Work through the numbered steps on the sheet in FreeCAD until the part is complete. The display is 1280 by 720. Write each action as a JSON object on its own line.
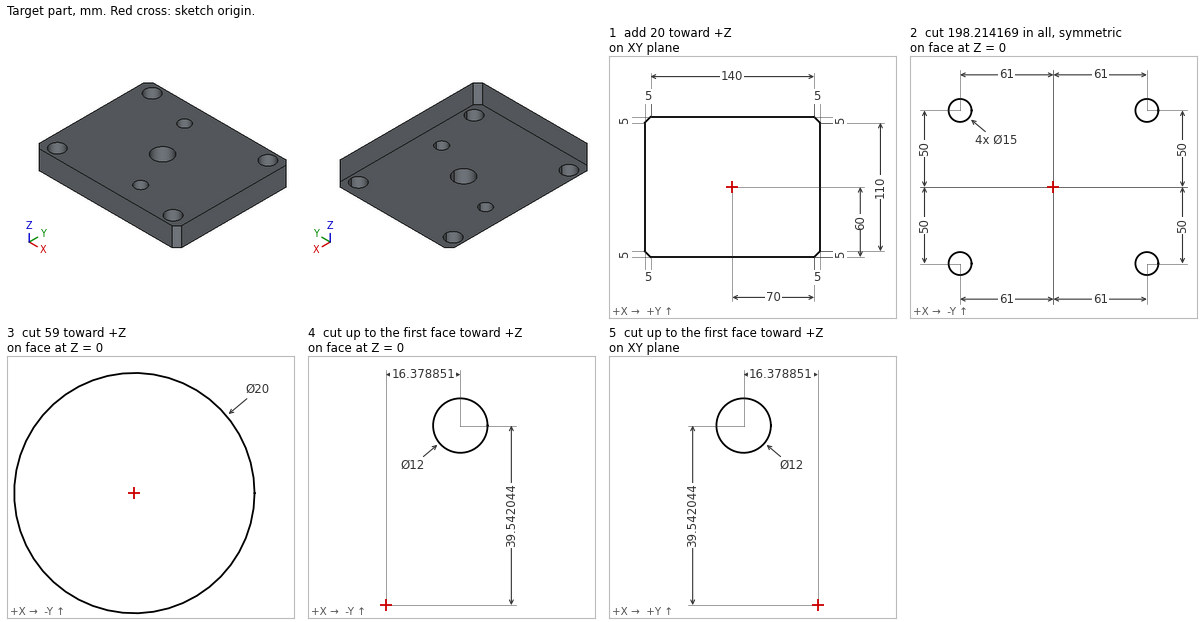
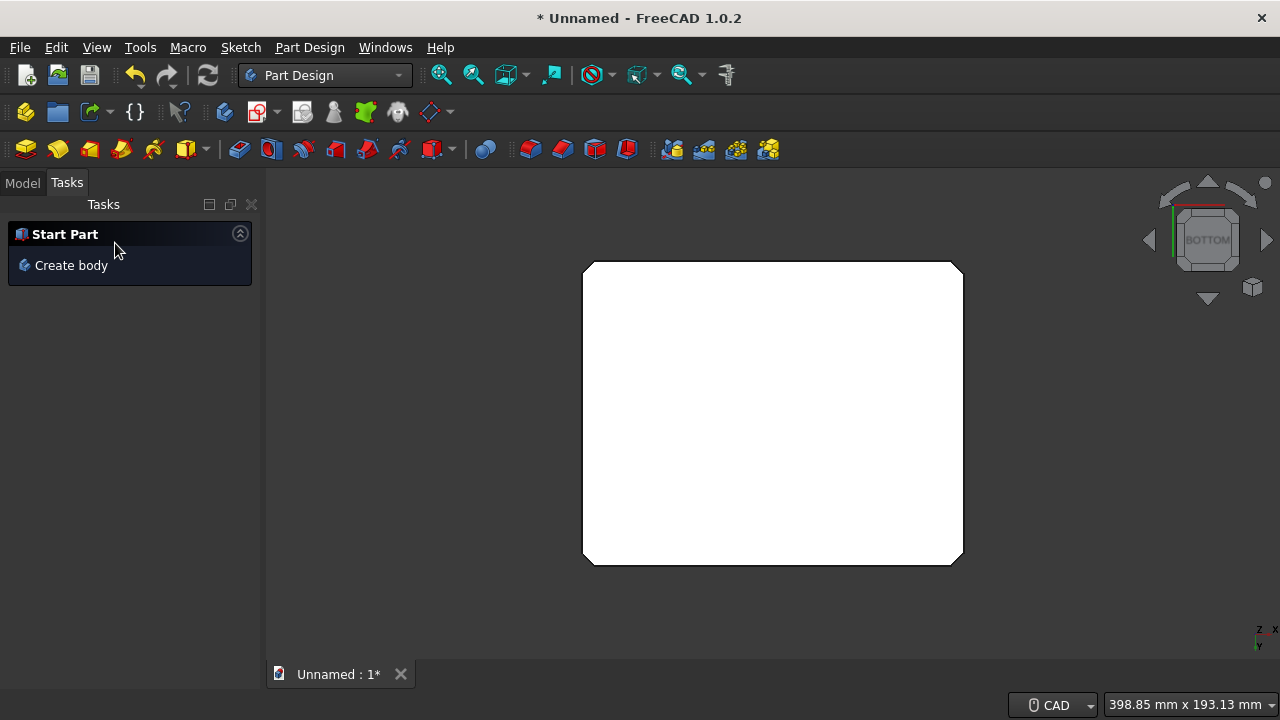
{"action": "left_click", "coordinate": [773, 412]}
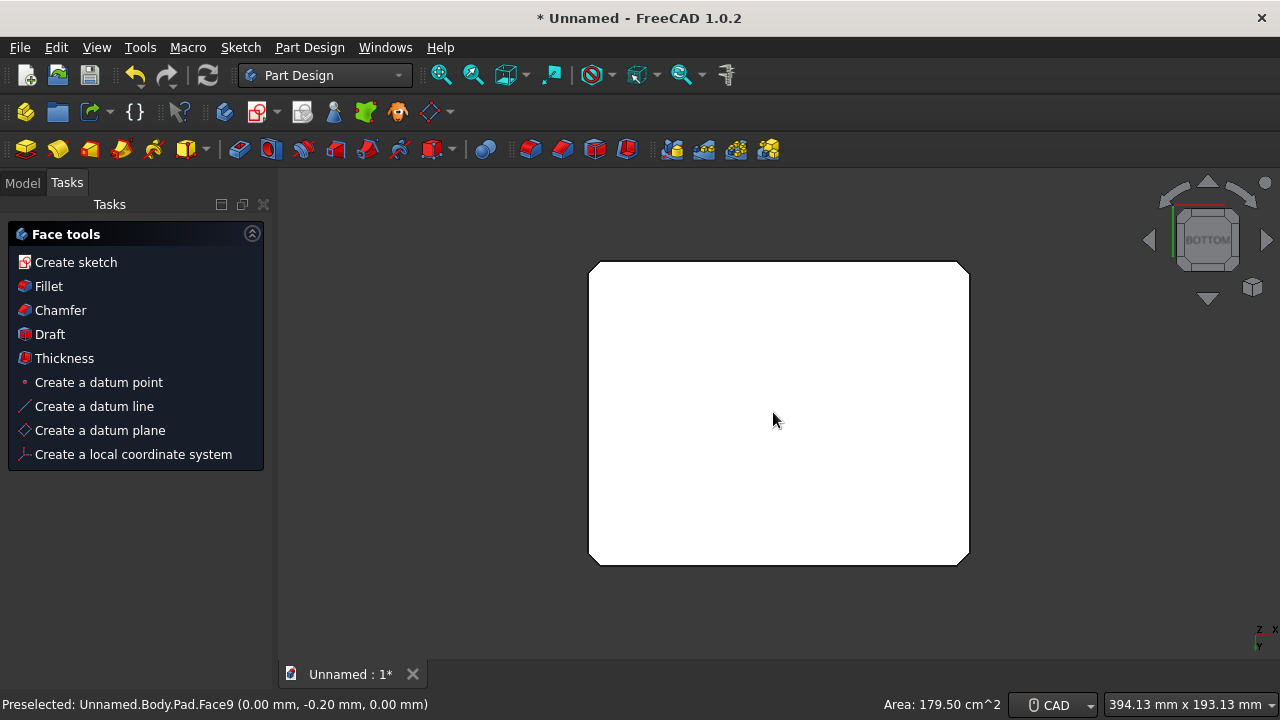
{"action": "left_click", "coordinate": [258, 112]}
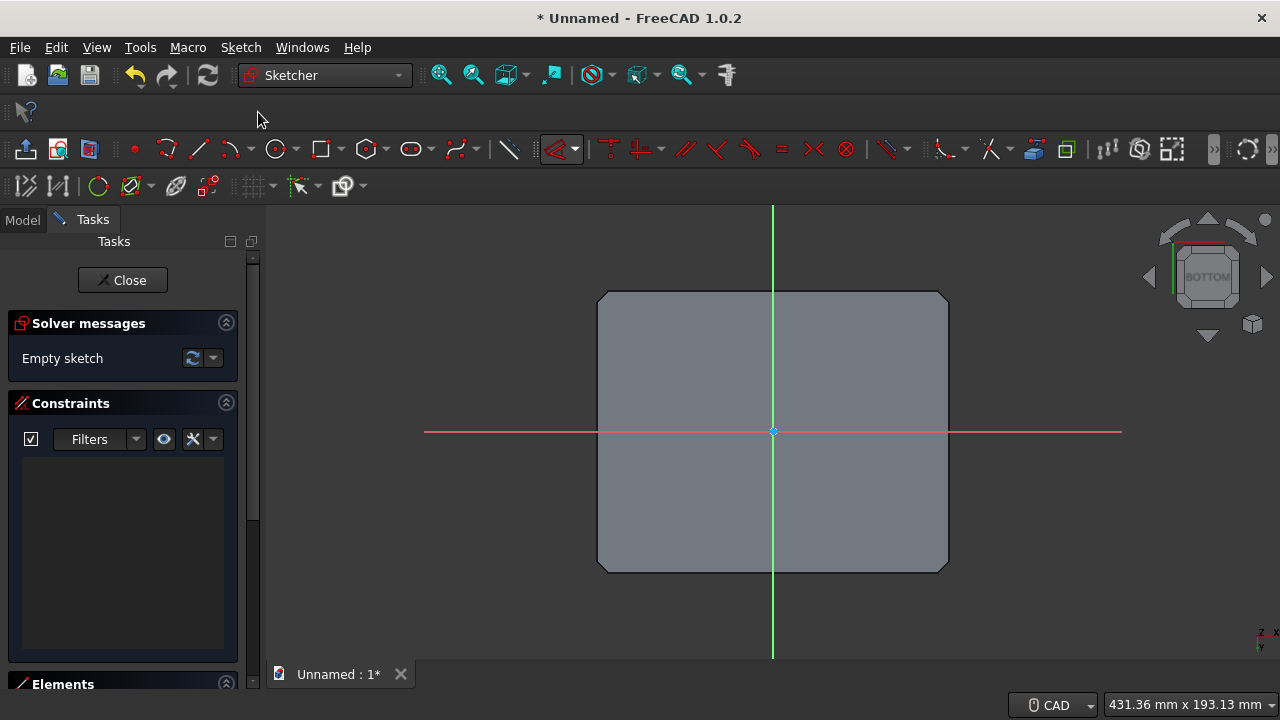
{"action": "key", "text": "g c"}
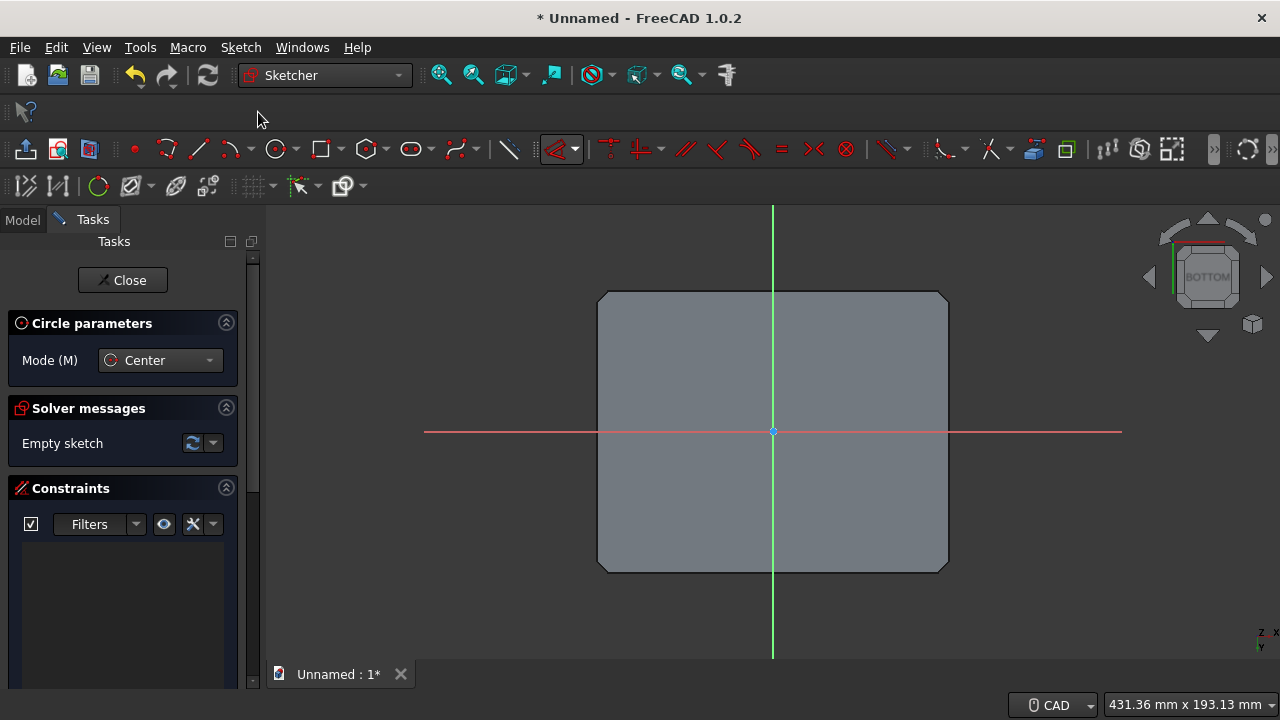
{"action": "scroll", "coordinate": [630, 314], "scroll_direction": "up", "scroll_amount": 2}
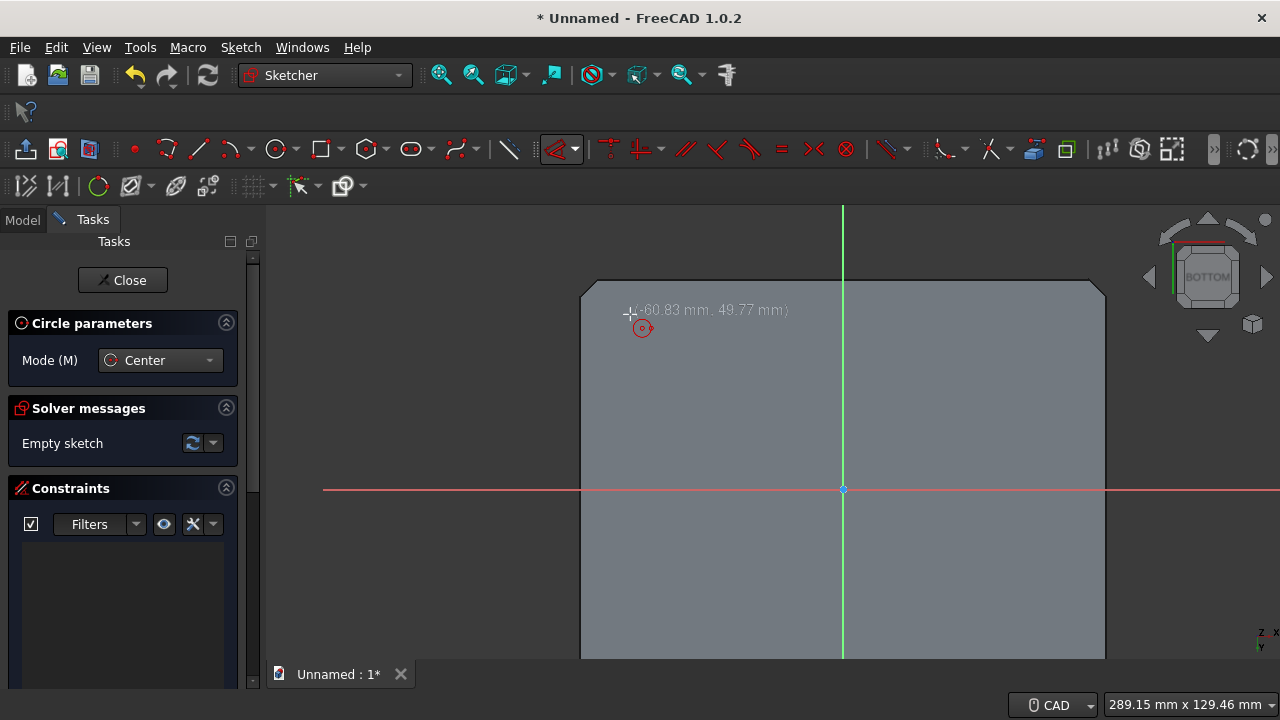
{"action": "left_click", "coordinate": [629, 315]}
{"action": "mouse_move", "coordinate": [648, 296]}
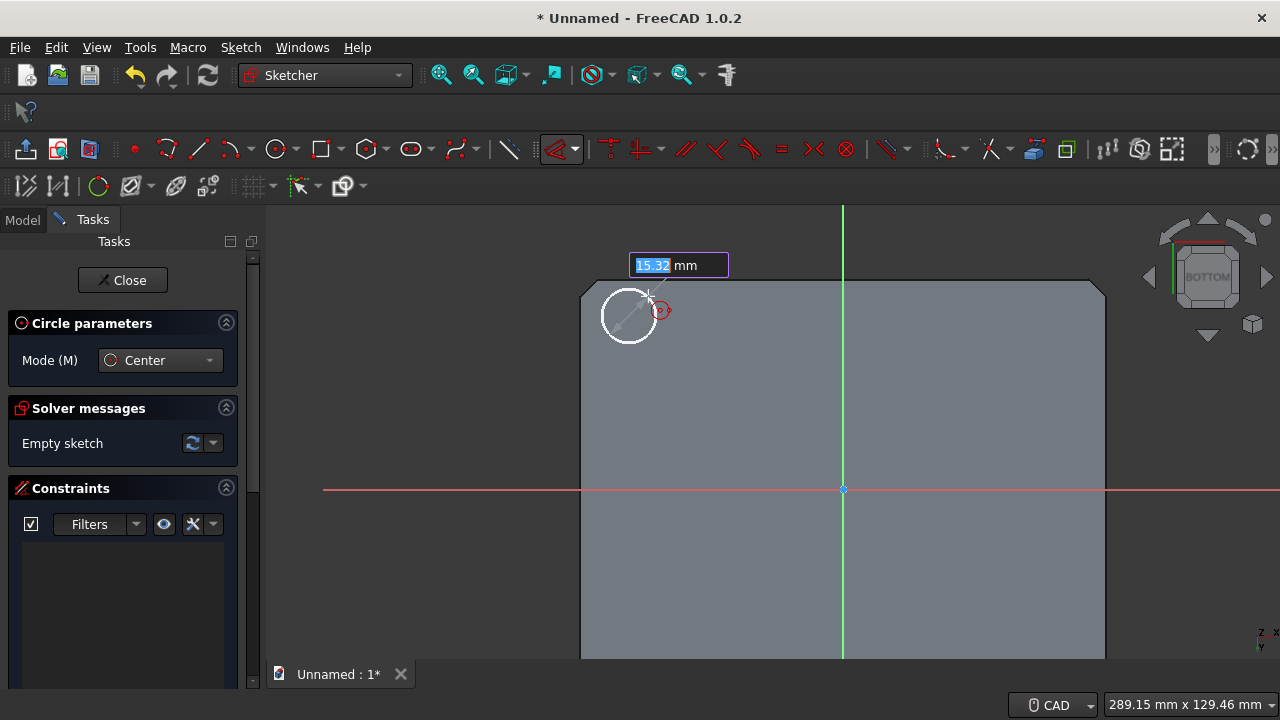
{"action": "type", "text": "15"}
{"action": "key", "text": "Return"}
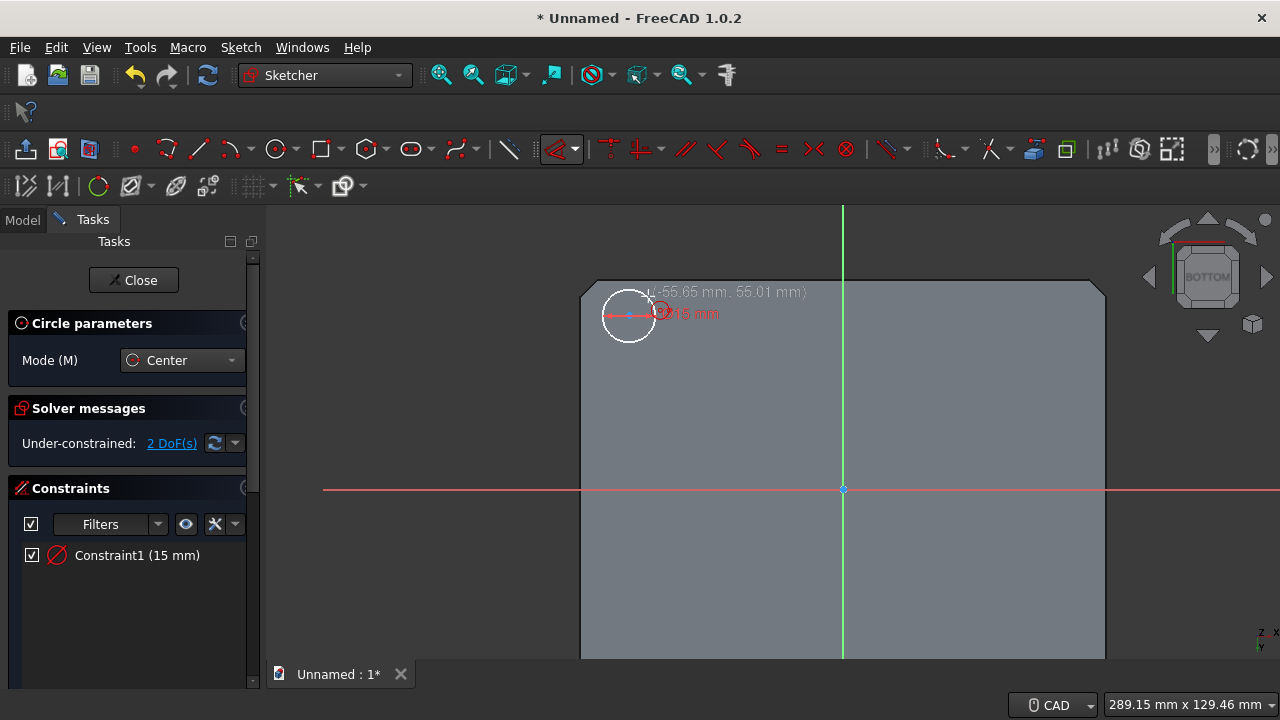
{"action": "scroll", "coordinate": [423, 314], "scroll_direction": "down", "scroll_amount": 2}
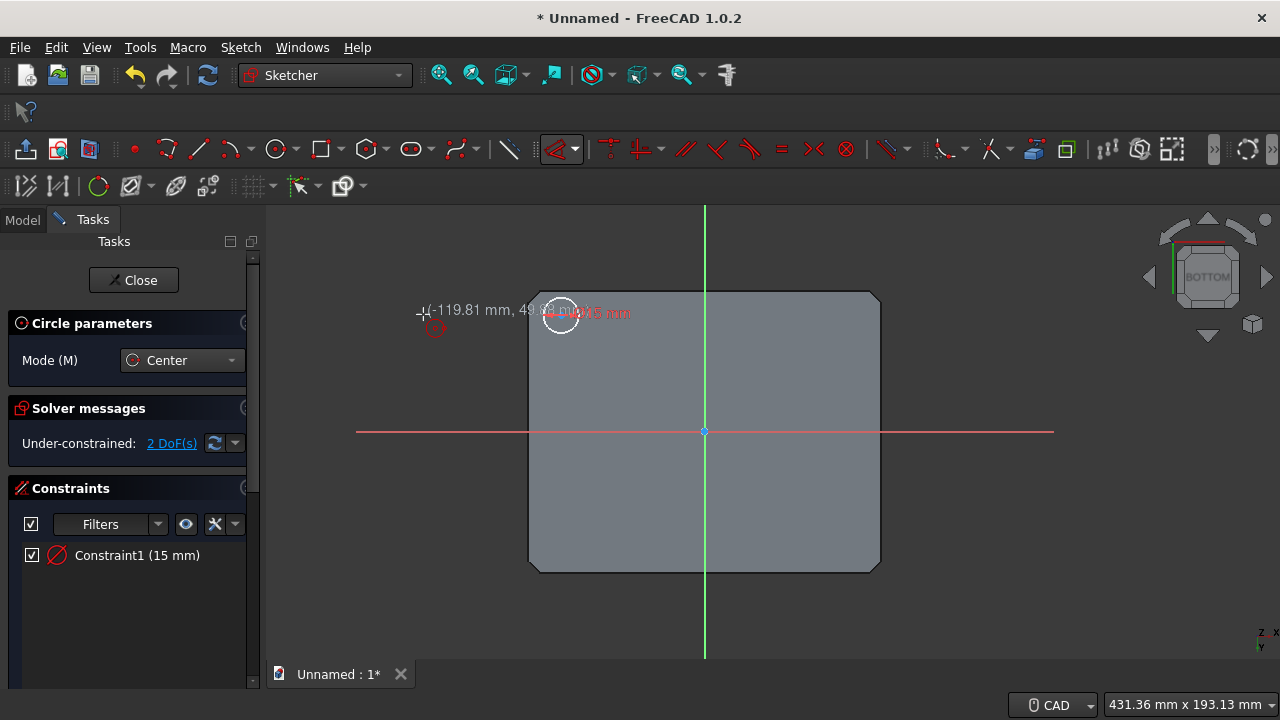
{"action": "scroll", "coordinate": [561, 550], "scroll_direction": "up", "scroll_amount": 2}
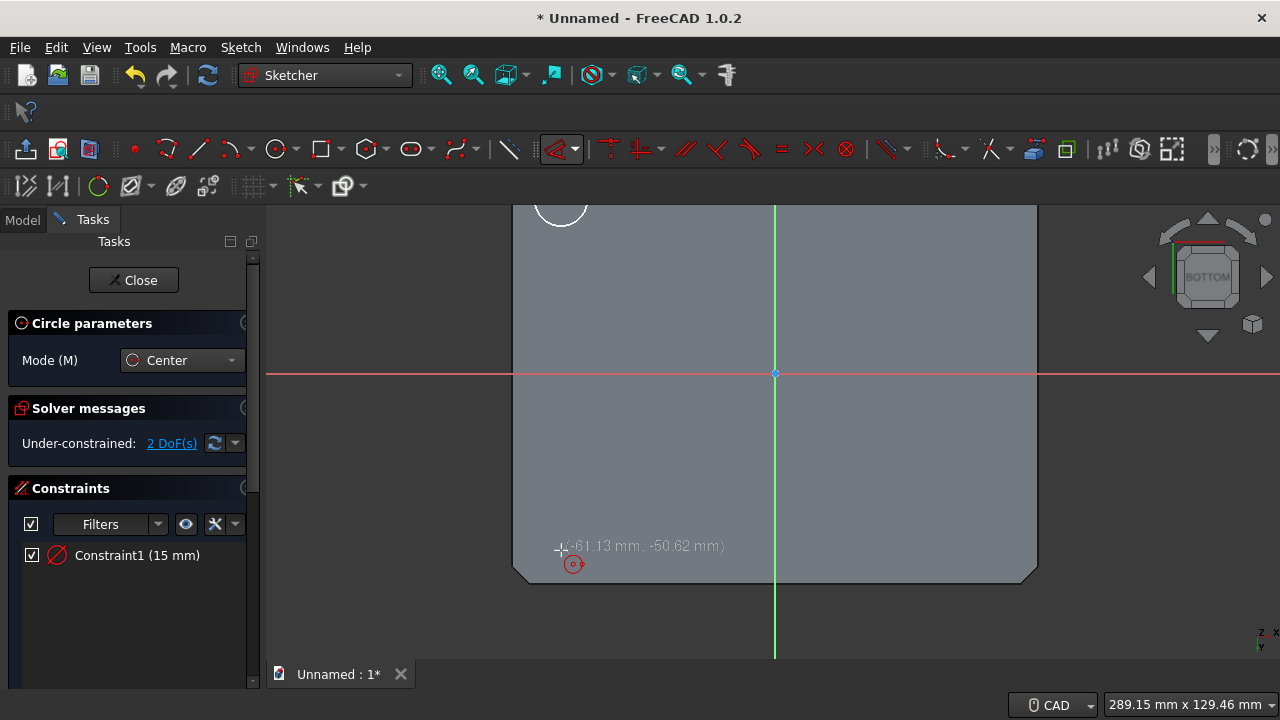
{"action": "left_click", "coordinate": [561, 549]}
{"action": "mouse_move", "coordinate": [580, 530]}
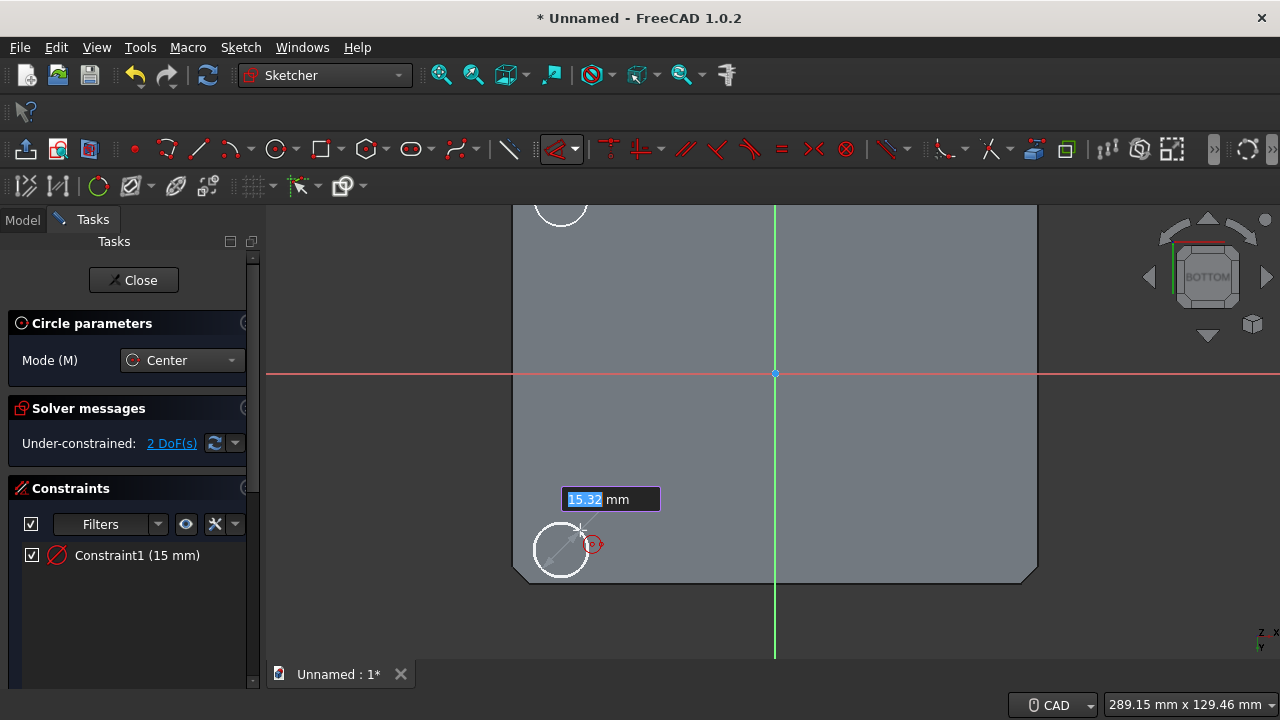
{"action": "type", "text": "15"}
{"action": "key", "text": "Return"}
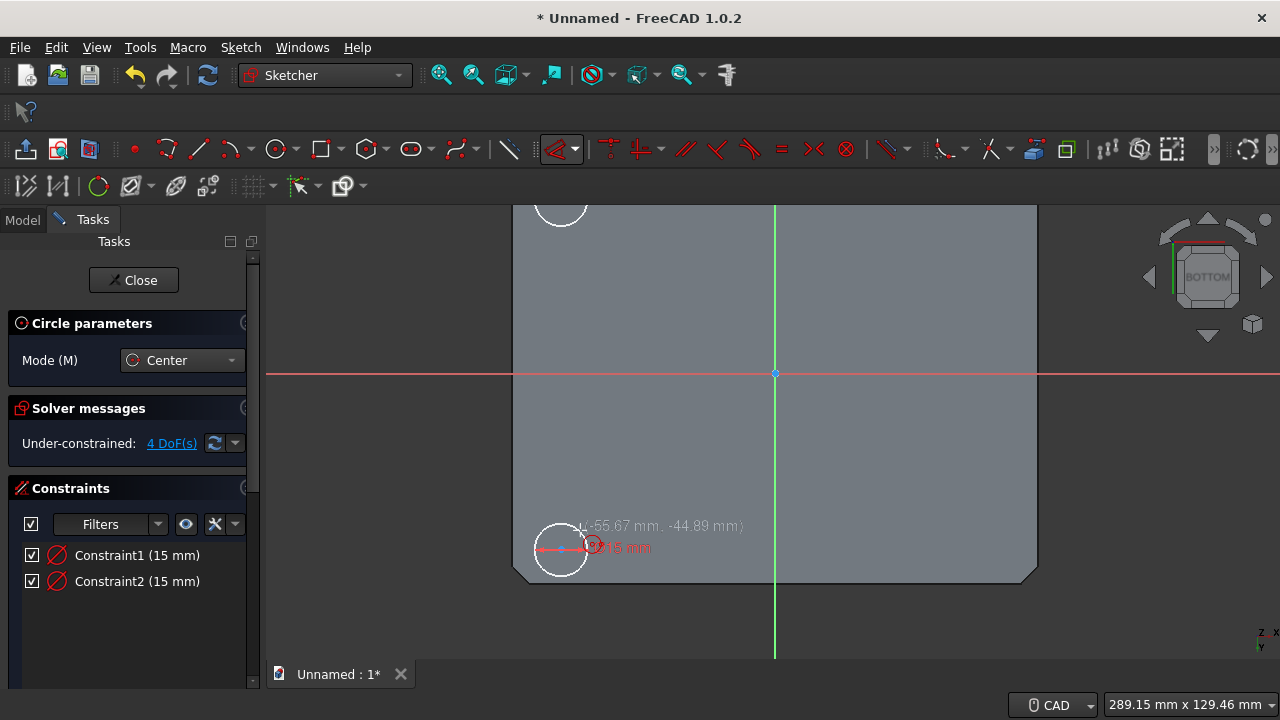
{"action": "scroll", "coordinate": [561, 551], "scroll_direction": "down", "scroll_amount": 2}